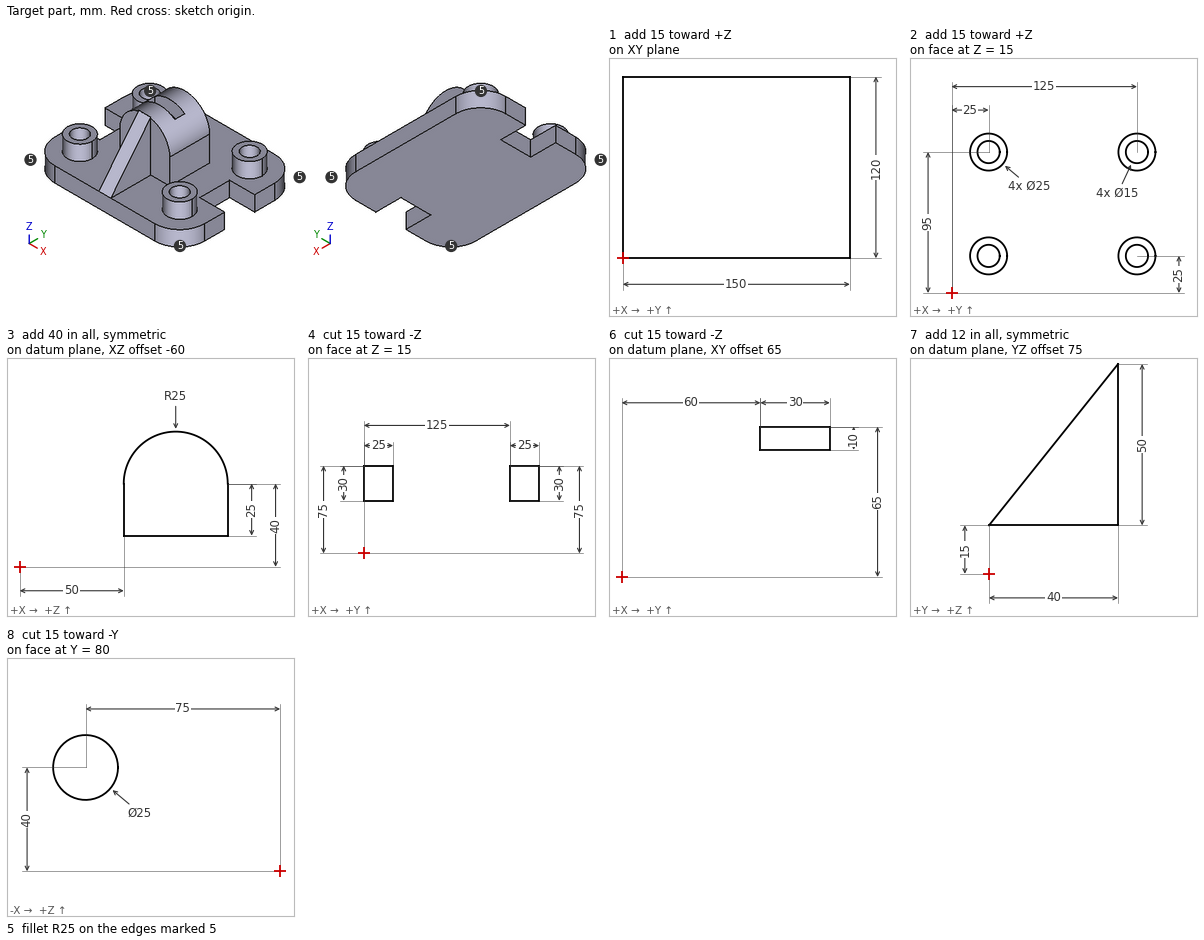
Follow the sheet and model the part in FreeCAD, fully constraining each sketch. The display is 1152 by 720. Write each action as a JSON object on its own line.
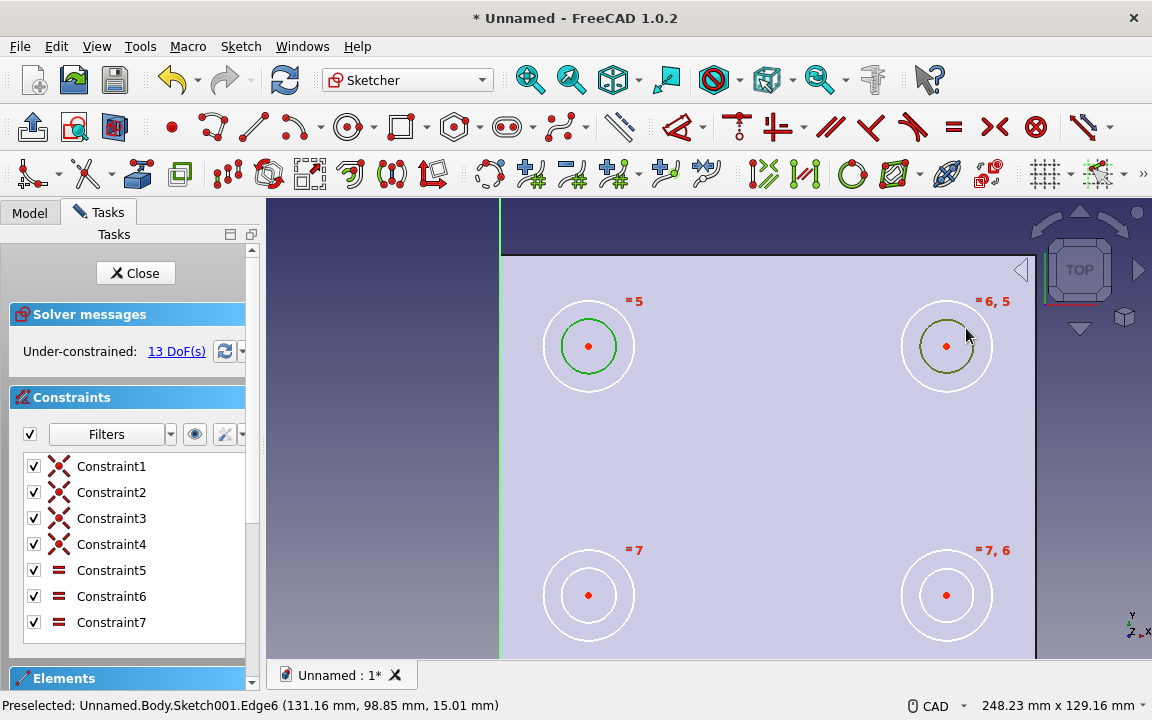
{"action": "left_click", "coordinate": [966, 577]}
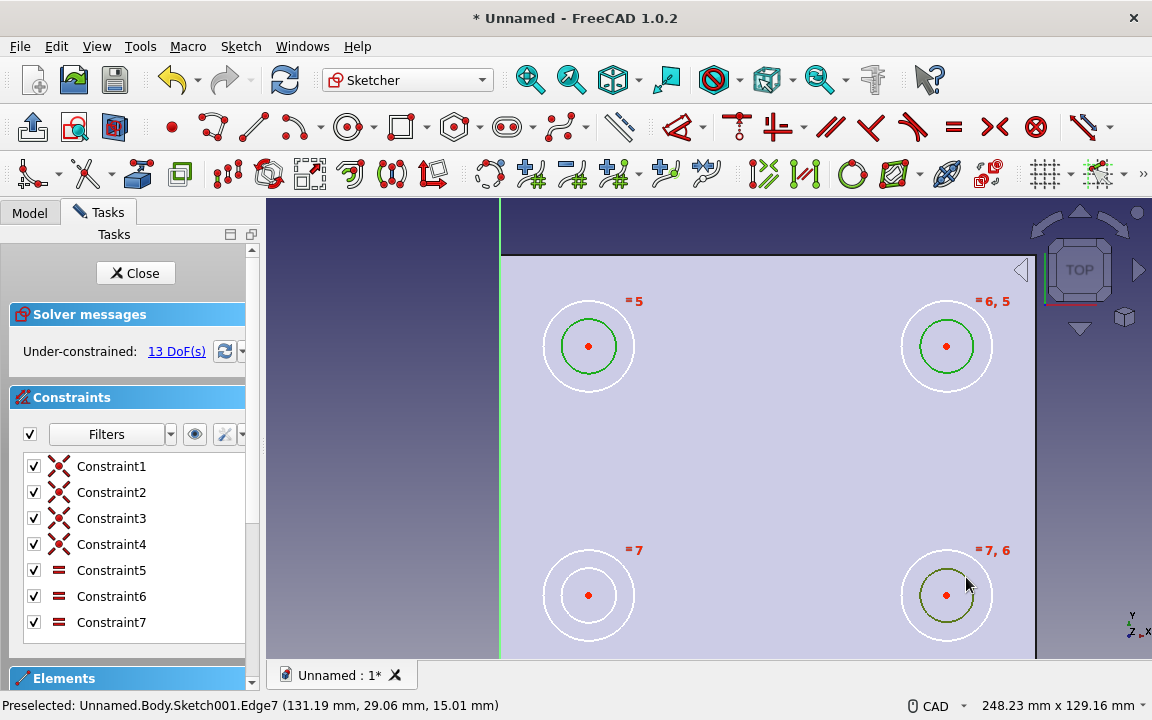
{"action": "left_click", "coordinate": [608, 576]}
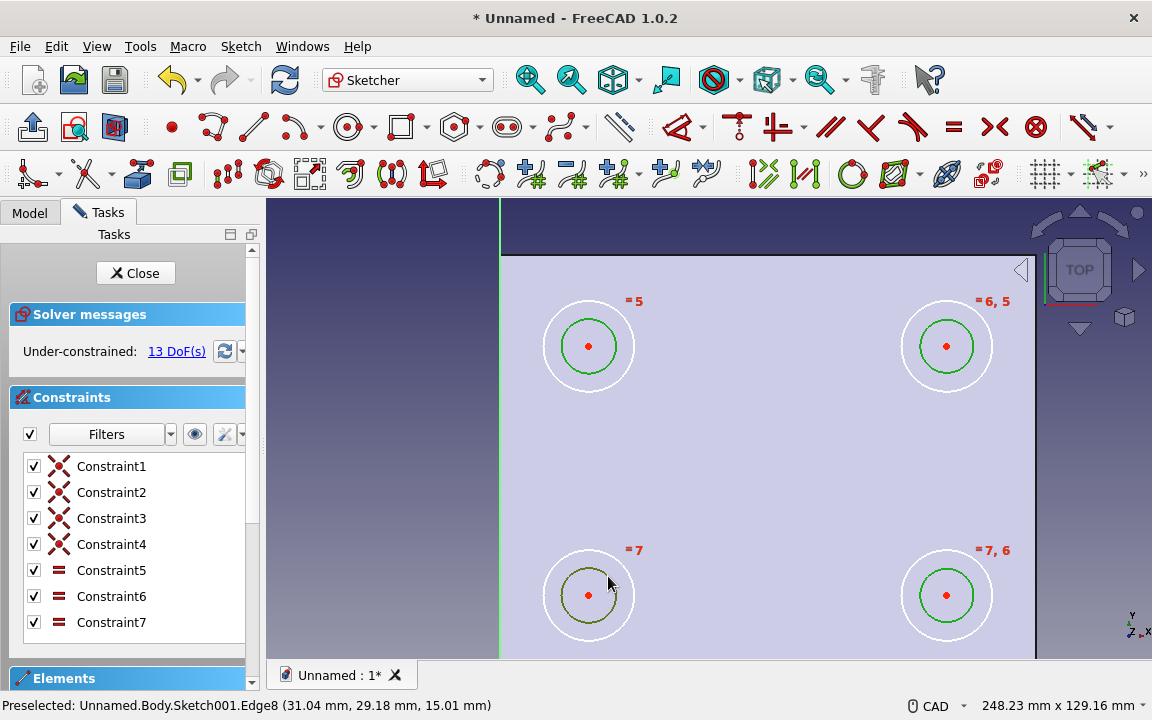
{"action": "left_click", "coordinate": [954, 128]}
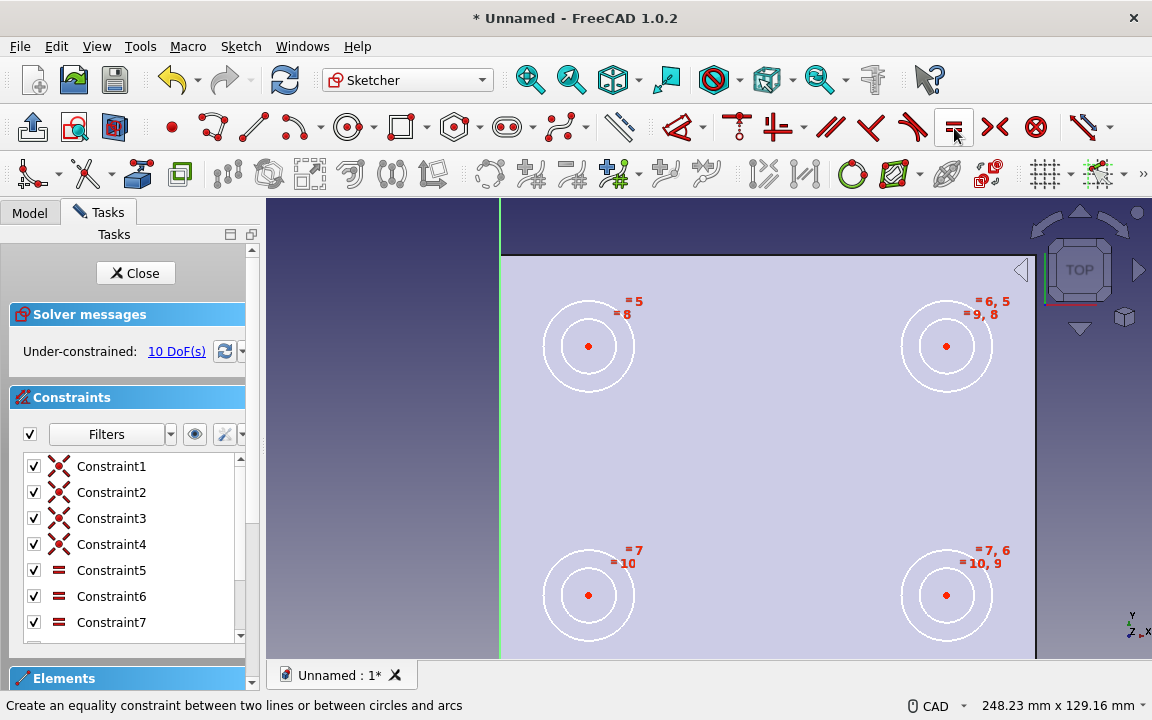
{"action": "left_click", "coordinate": [589, 346]}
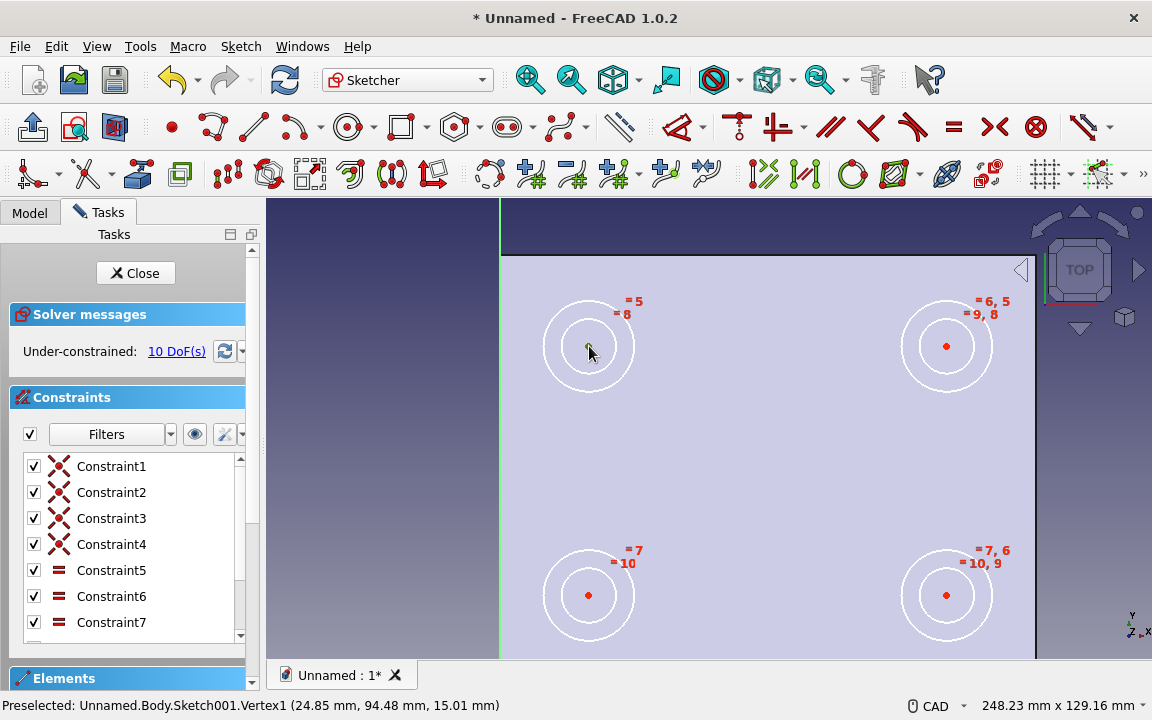
{"action": "left_click", "coordinate": [947, 346]}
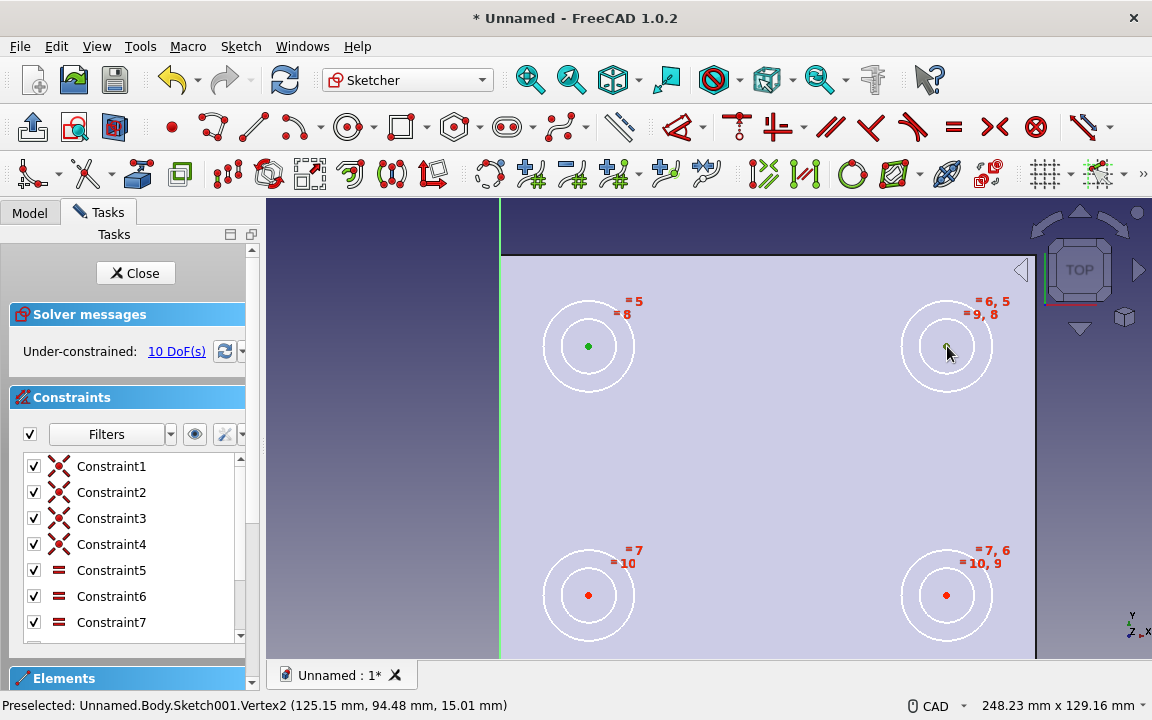
{"action": "key", "text": "h"}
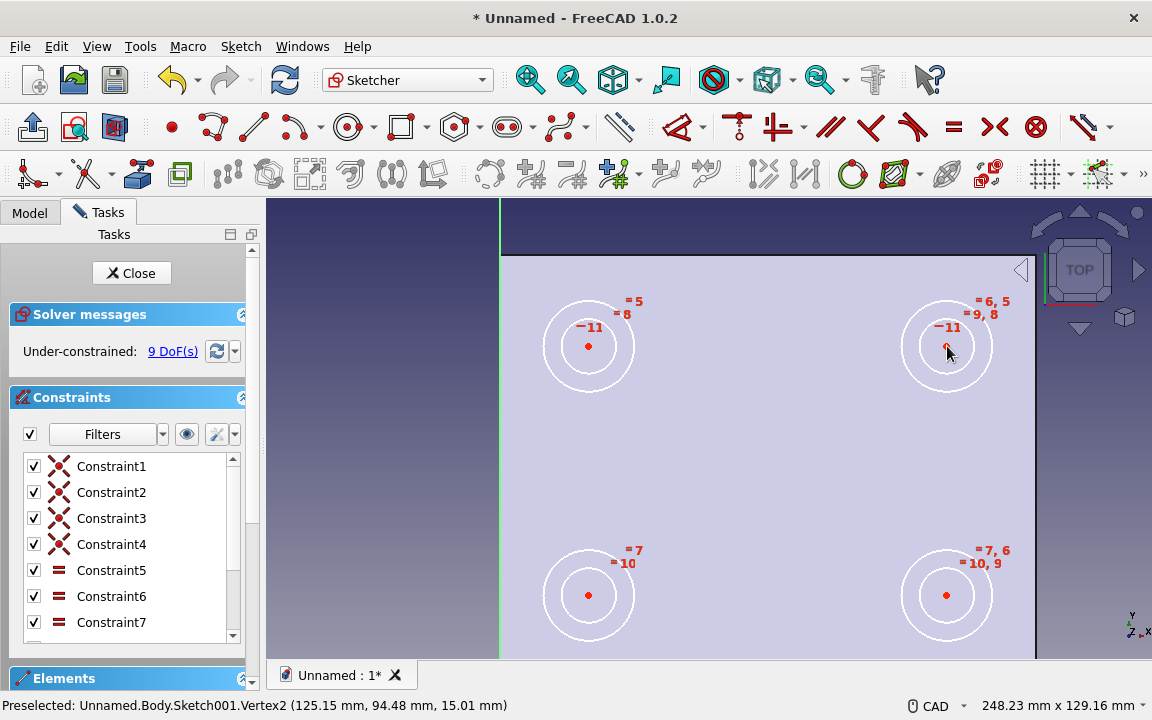
{"action": "left_click", "coordinate": [947, 346]}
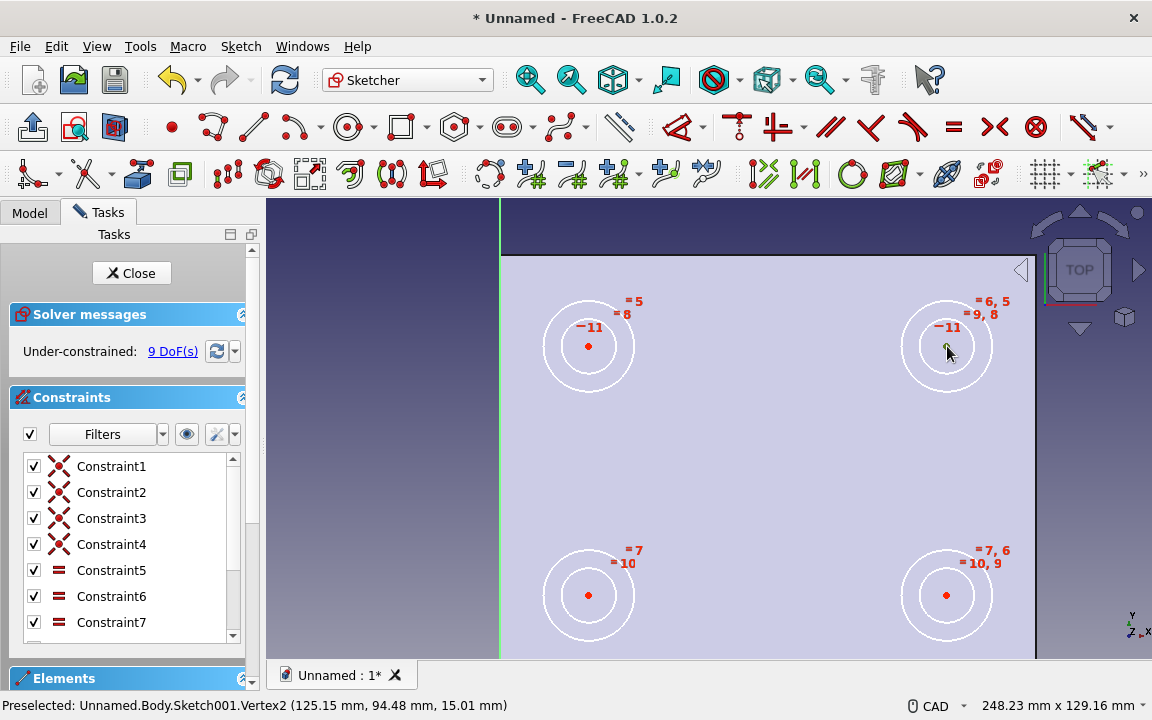
{"action": "left_click", "coordinate": [947, 595]}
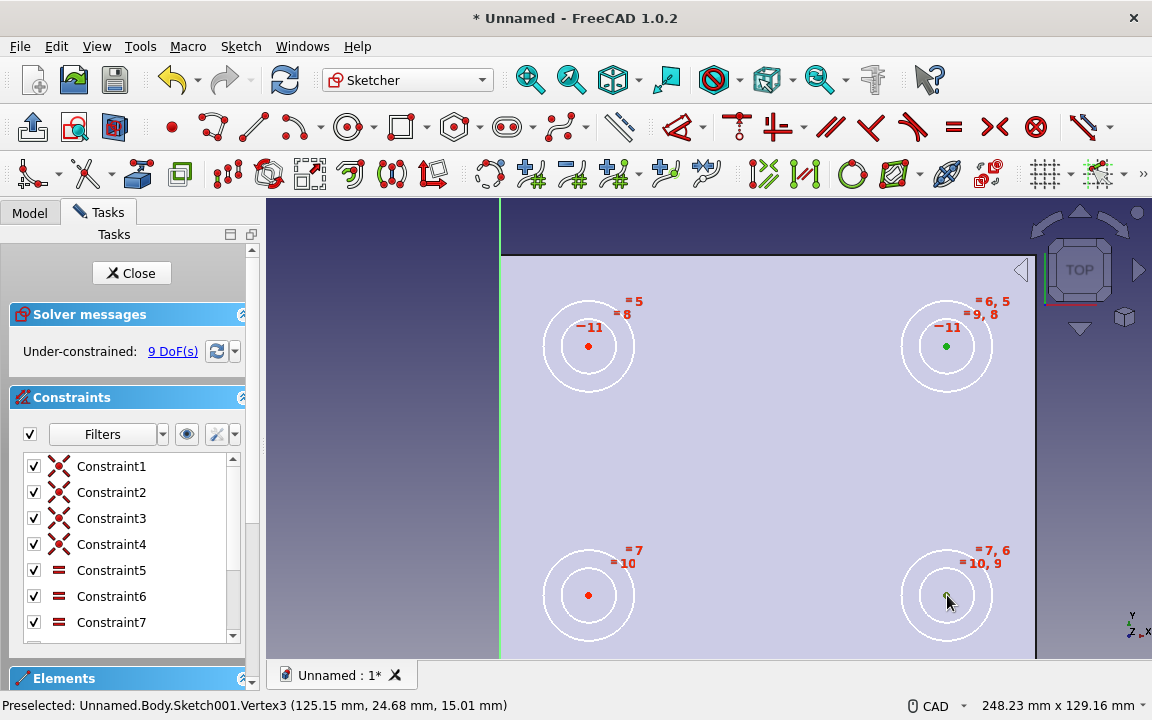
{"action": "left_click", "coordinate": [804, 128]}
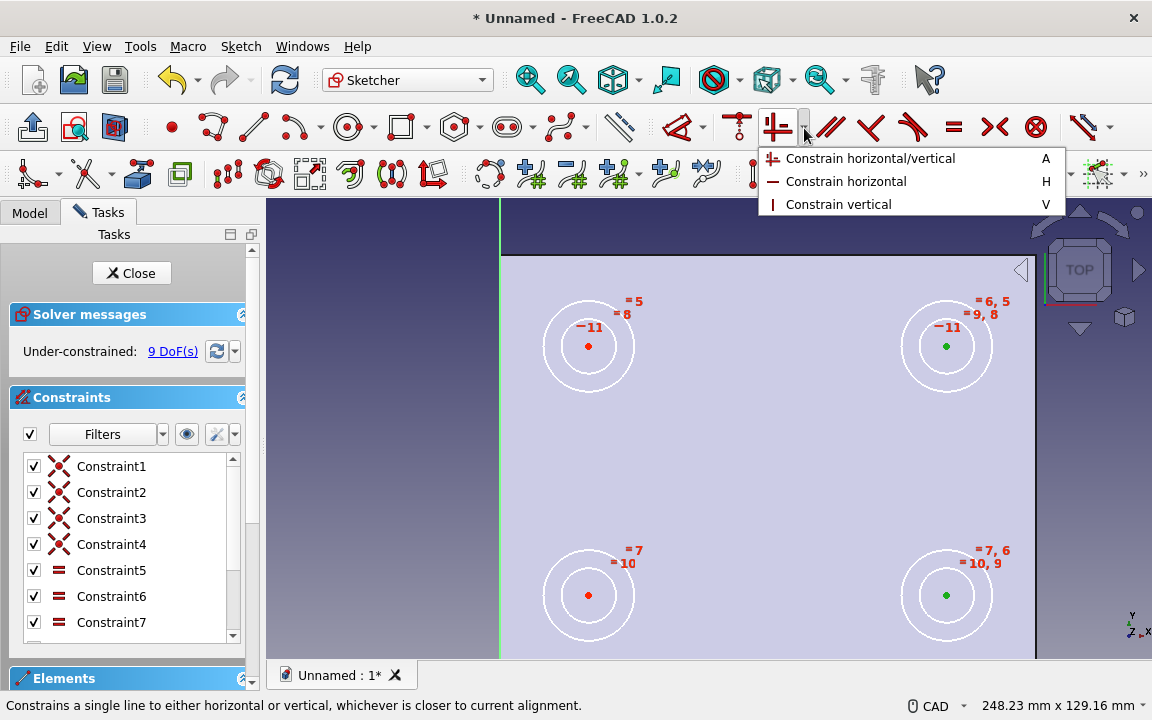
{"action": "left_click", "coordinate": [912, 204]}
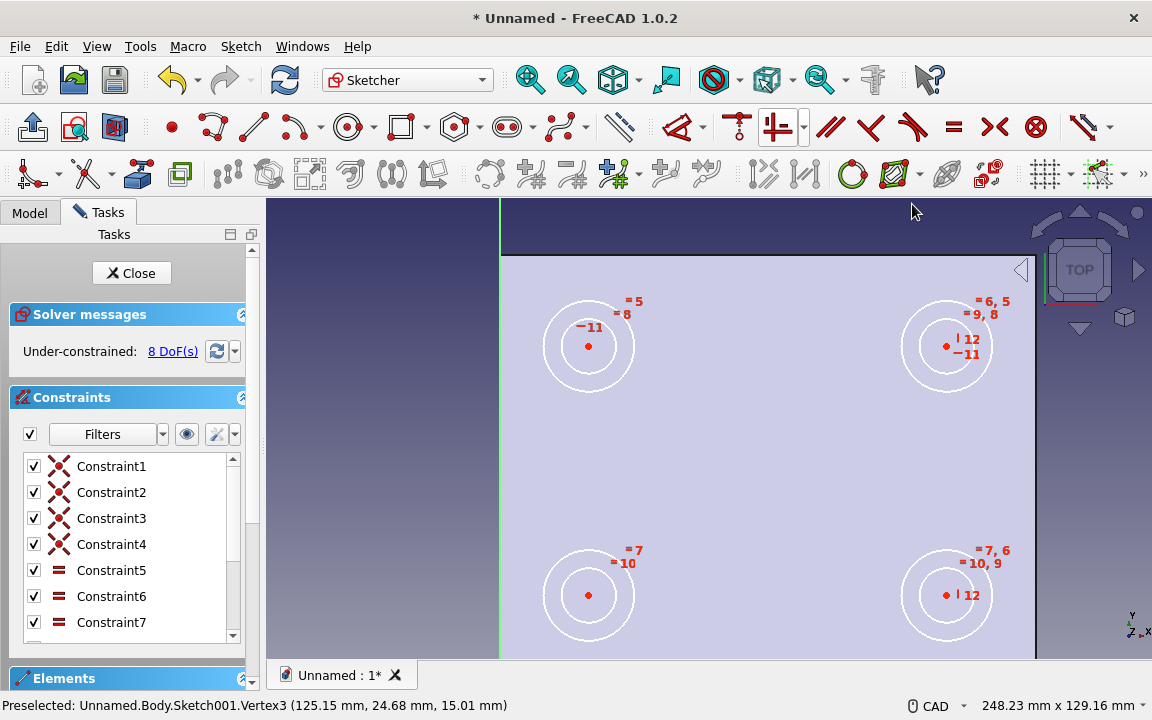
{"action": "left_click", "coordinate": [589, 346]}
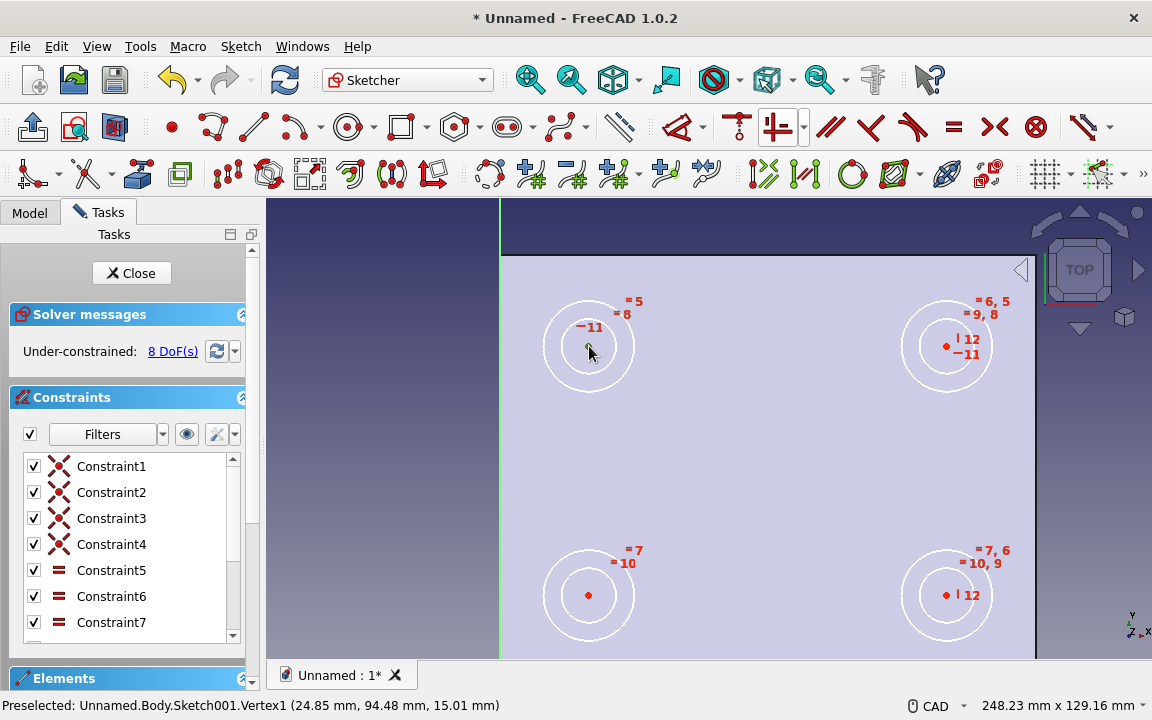
{"action": "left_click", "coordinate": [589, 595]}